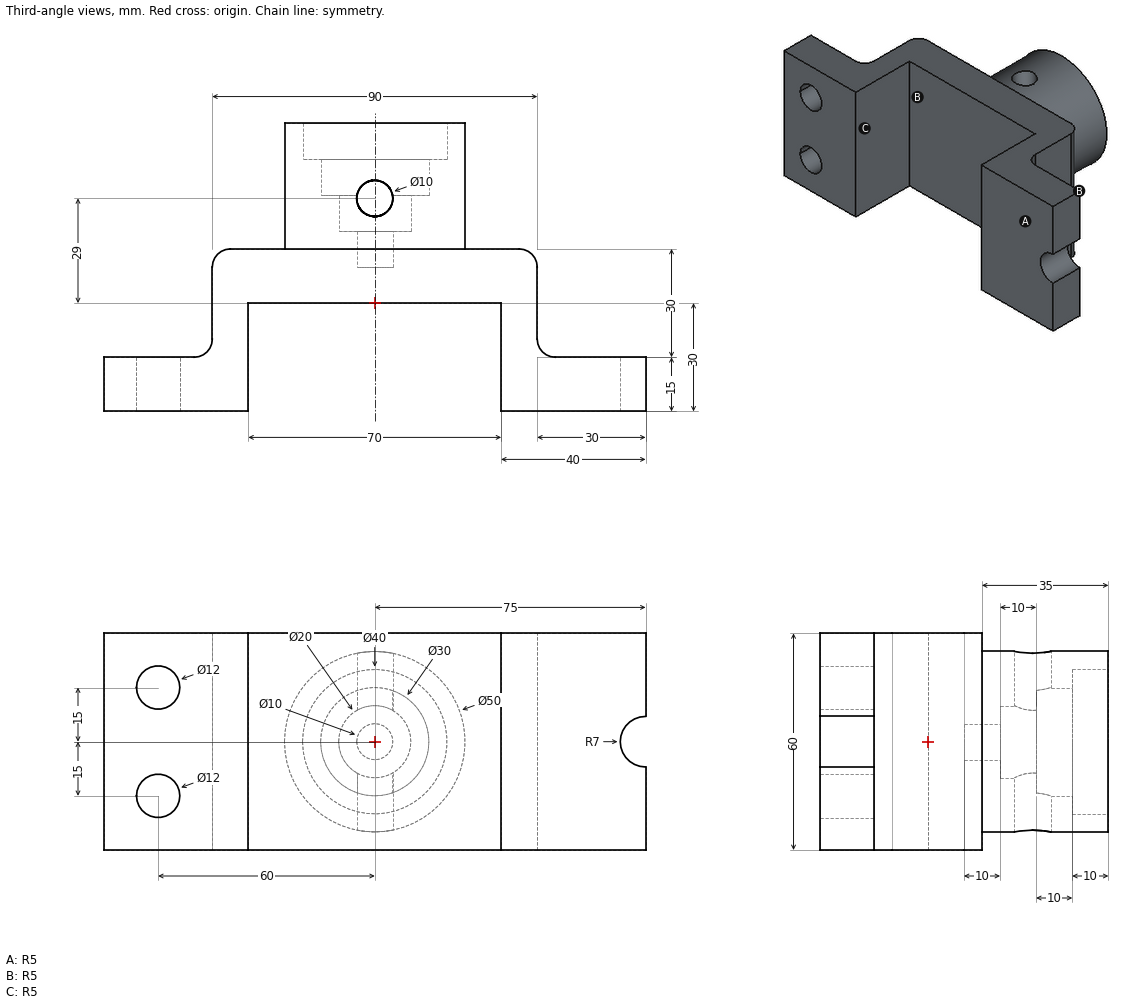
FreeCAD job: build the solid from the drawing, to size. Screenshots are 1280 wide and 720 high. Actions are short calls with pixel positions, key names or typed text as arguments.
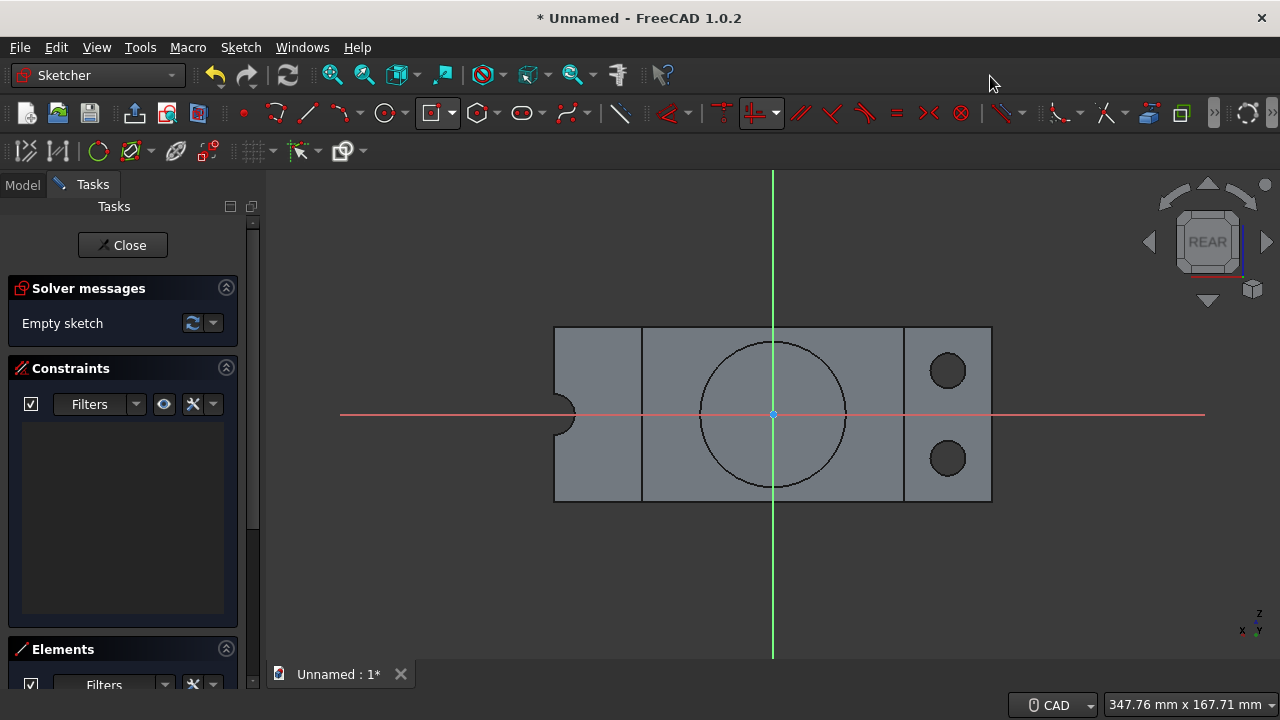
scroll(813, 415, up, 5)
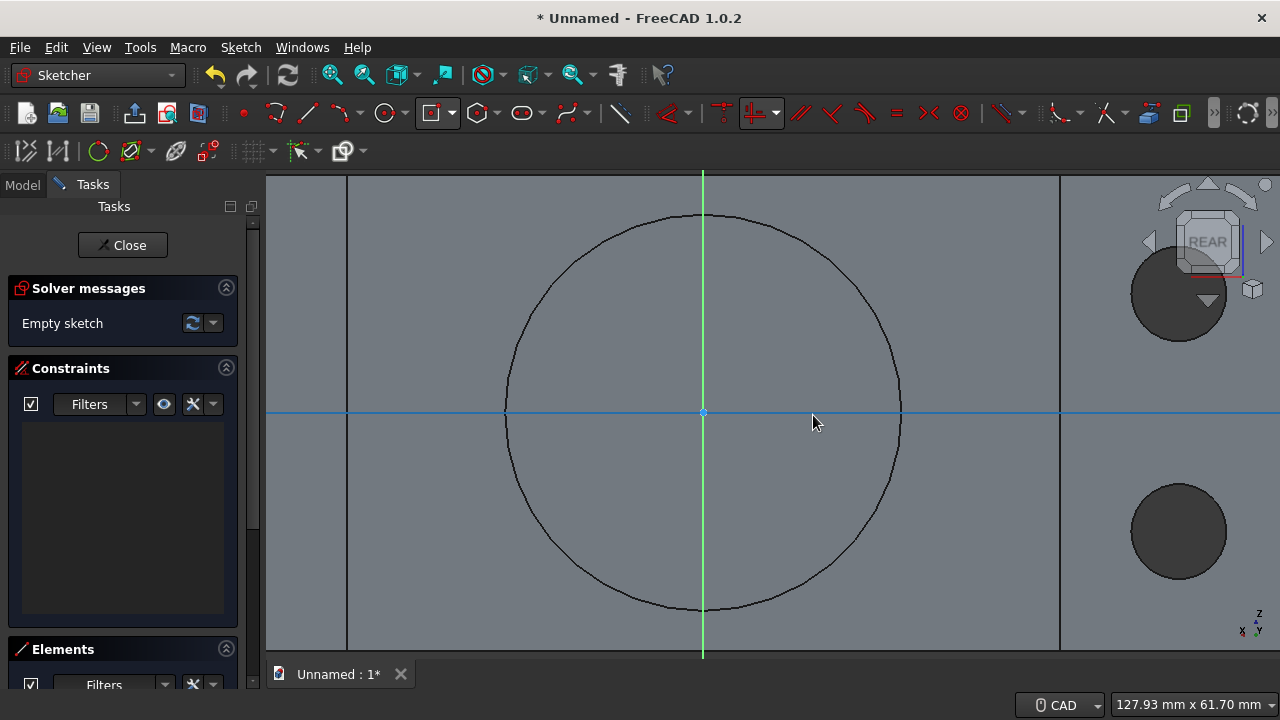
click(386, 114)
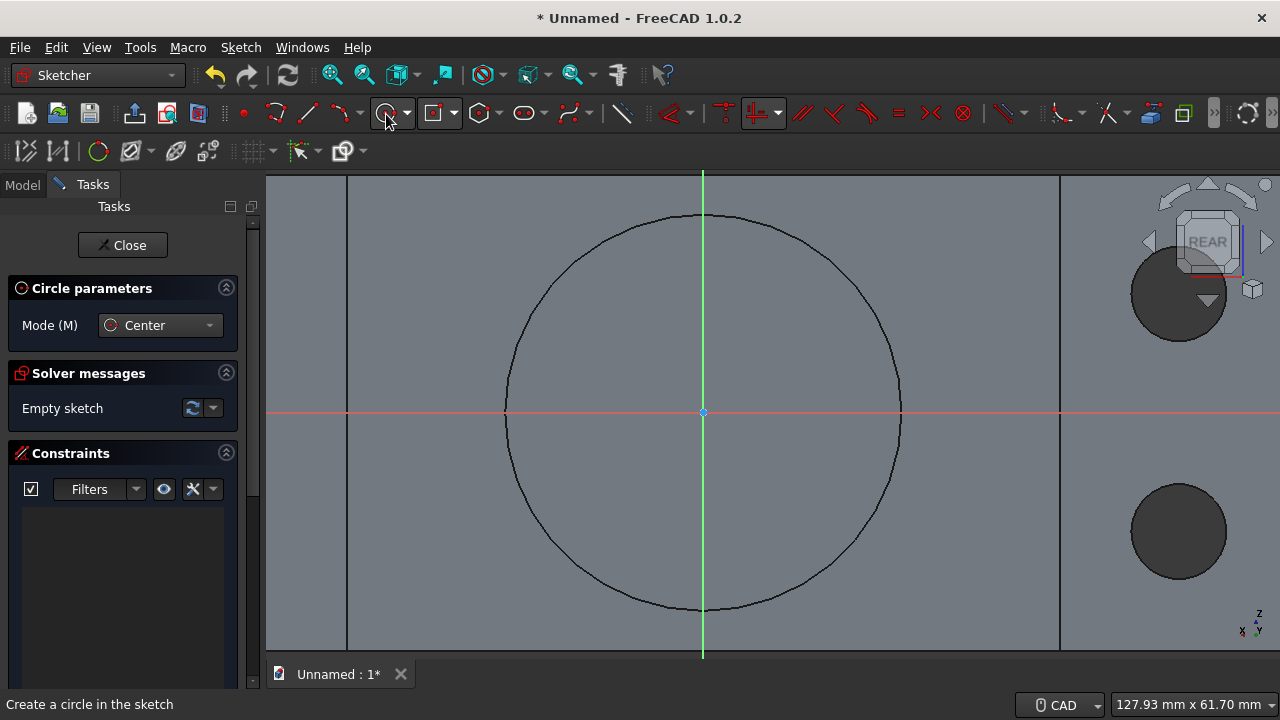
click(703, 413)
click(815, 301)
key(Escape)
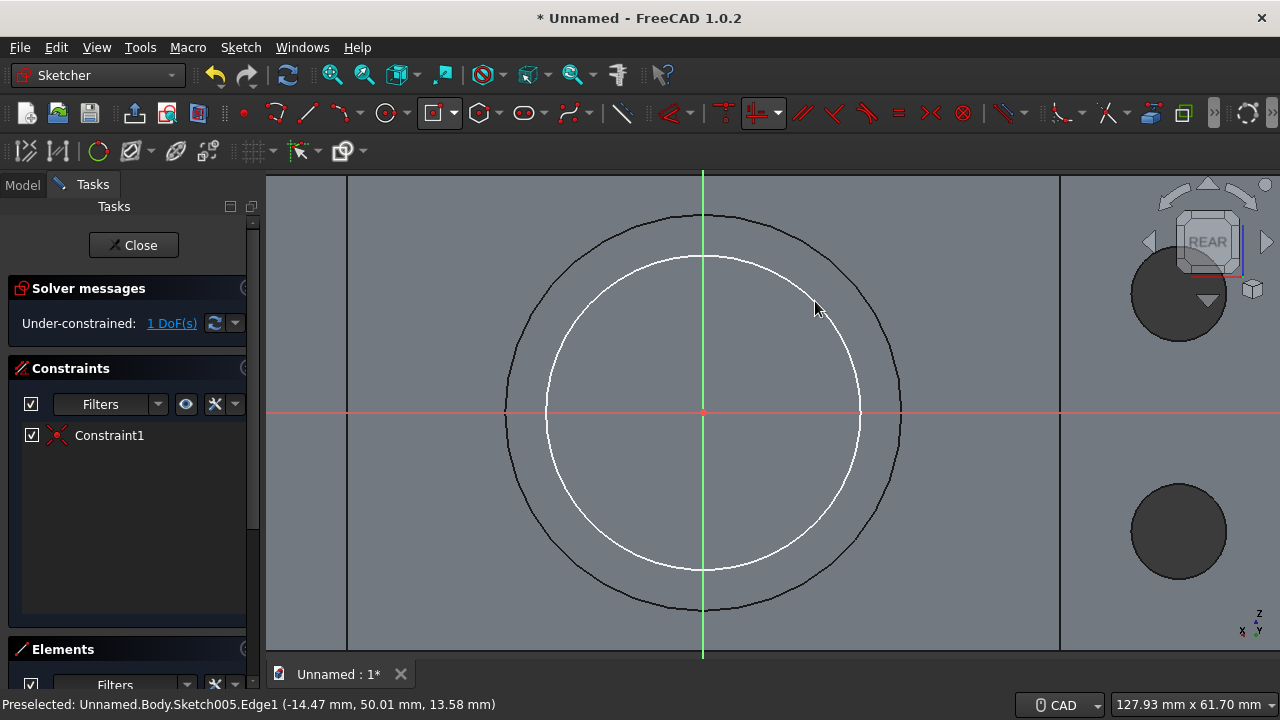
click(670, 114)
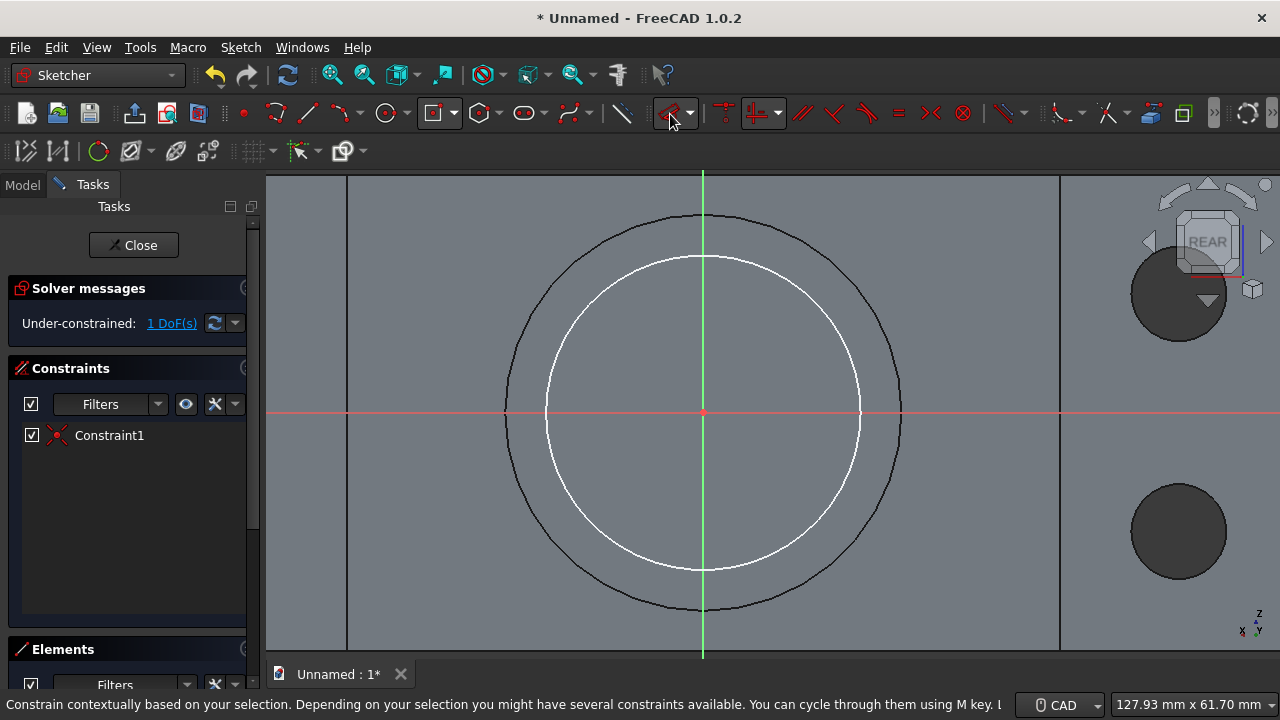
click(814, 301)
click(837, 278)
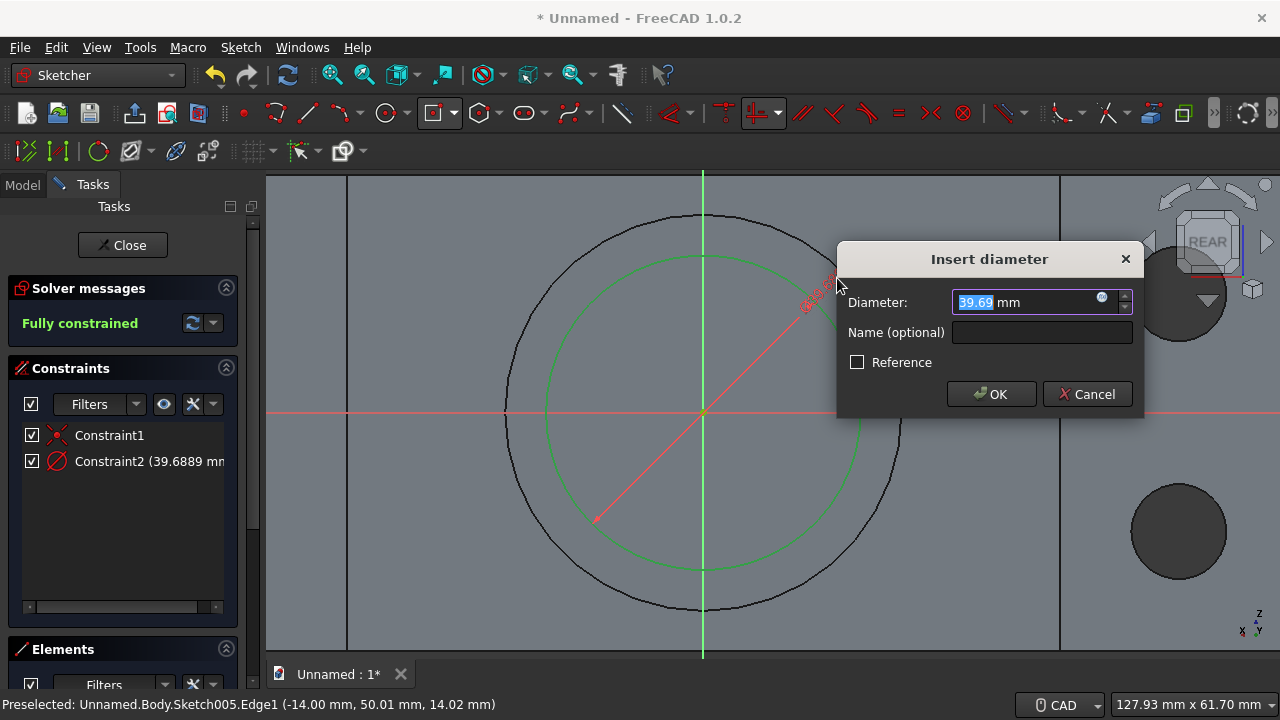
text(40)
key(Return)
key(Escape)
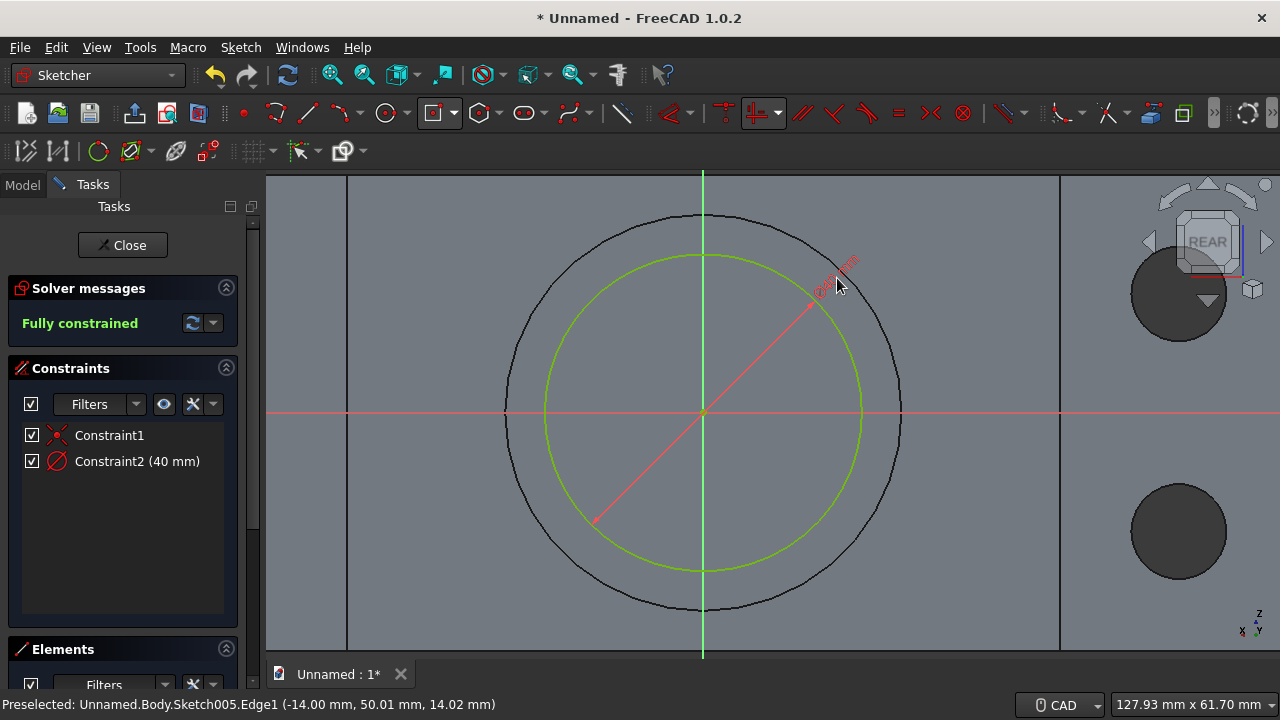
click(123, 245)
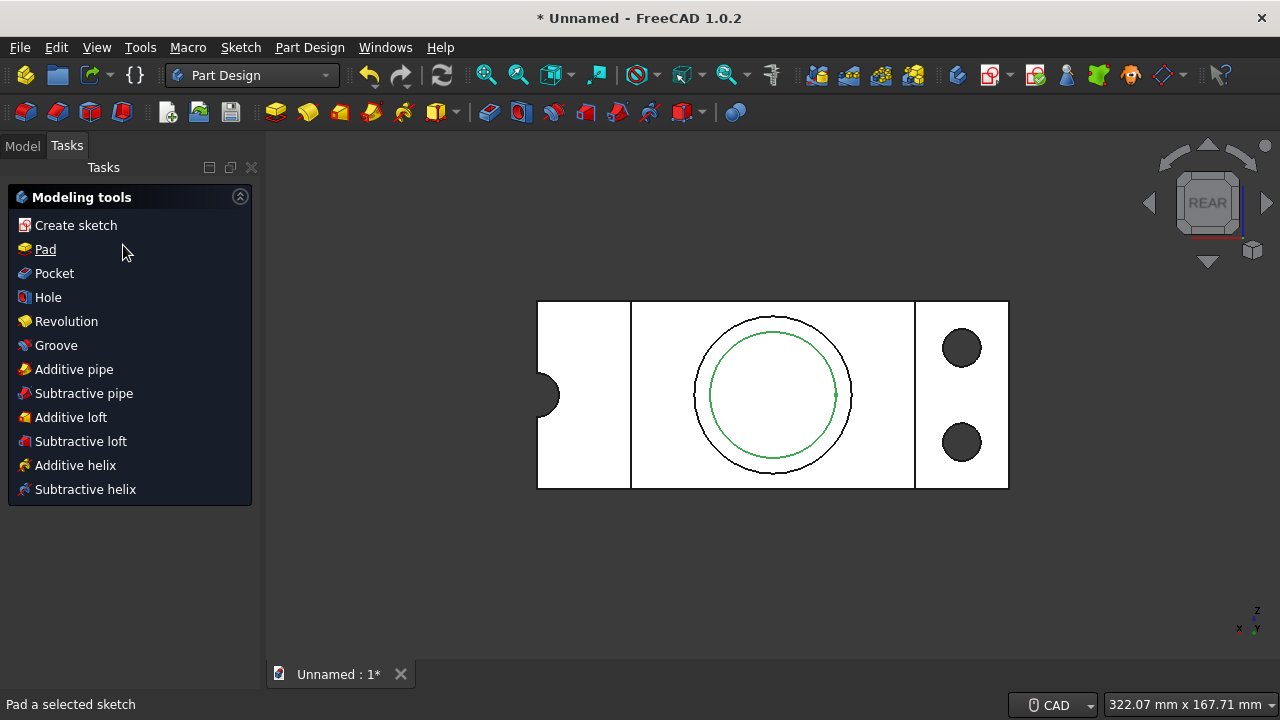
click(490, 112)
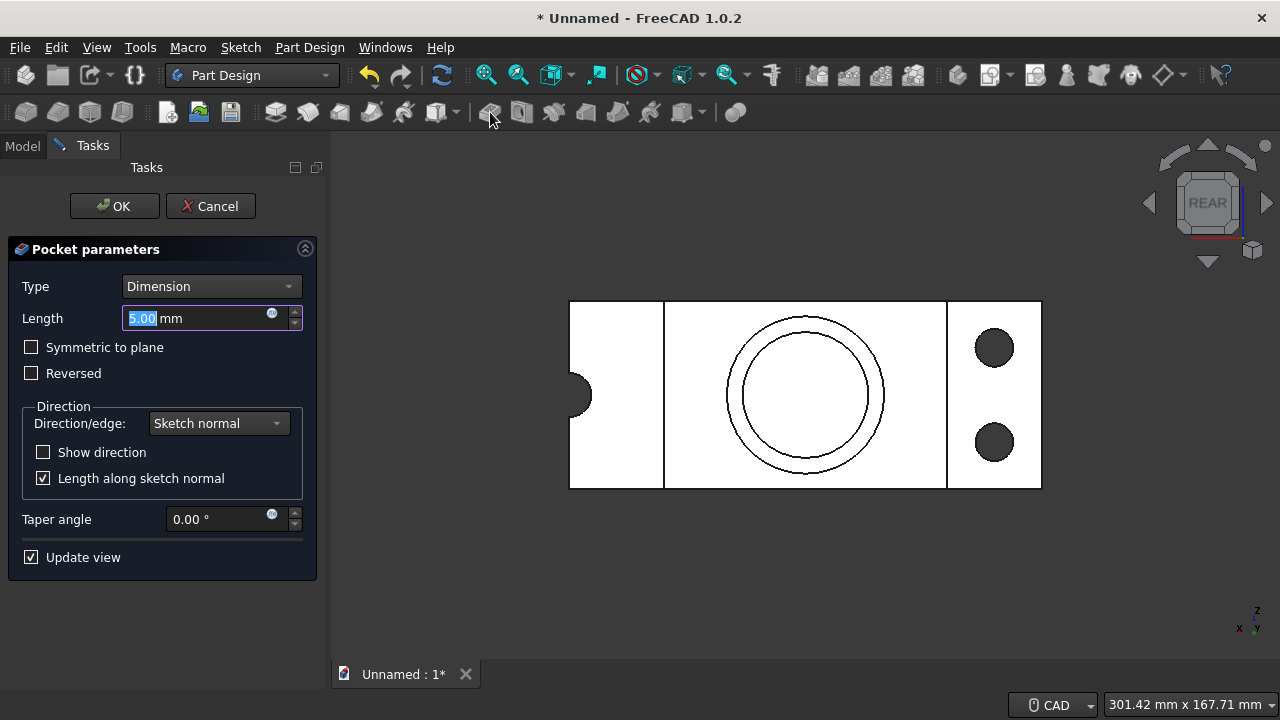
text(10)
key(Tab)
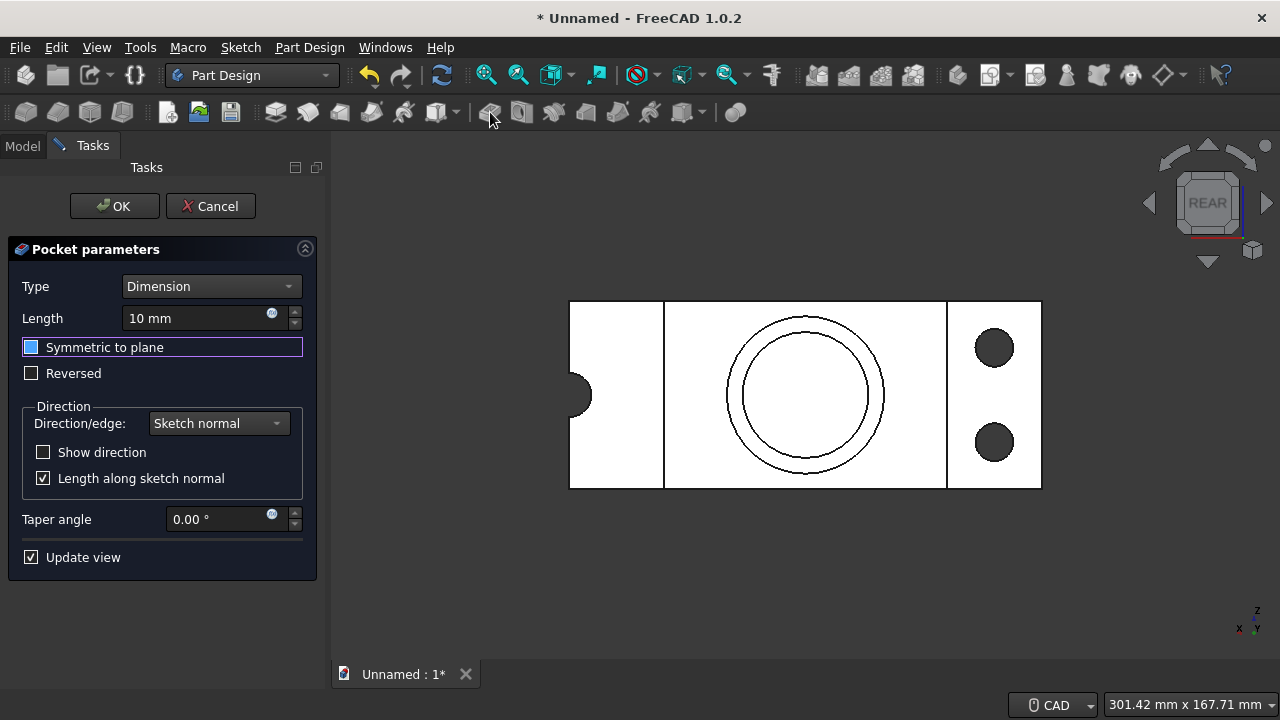
click(115, 206)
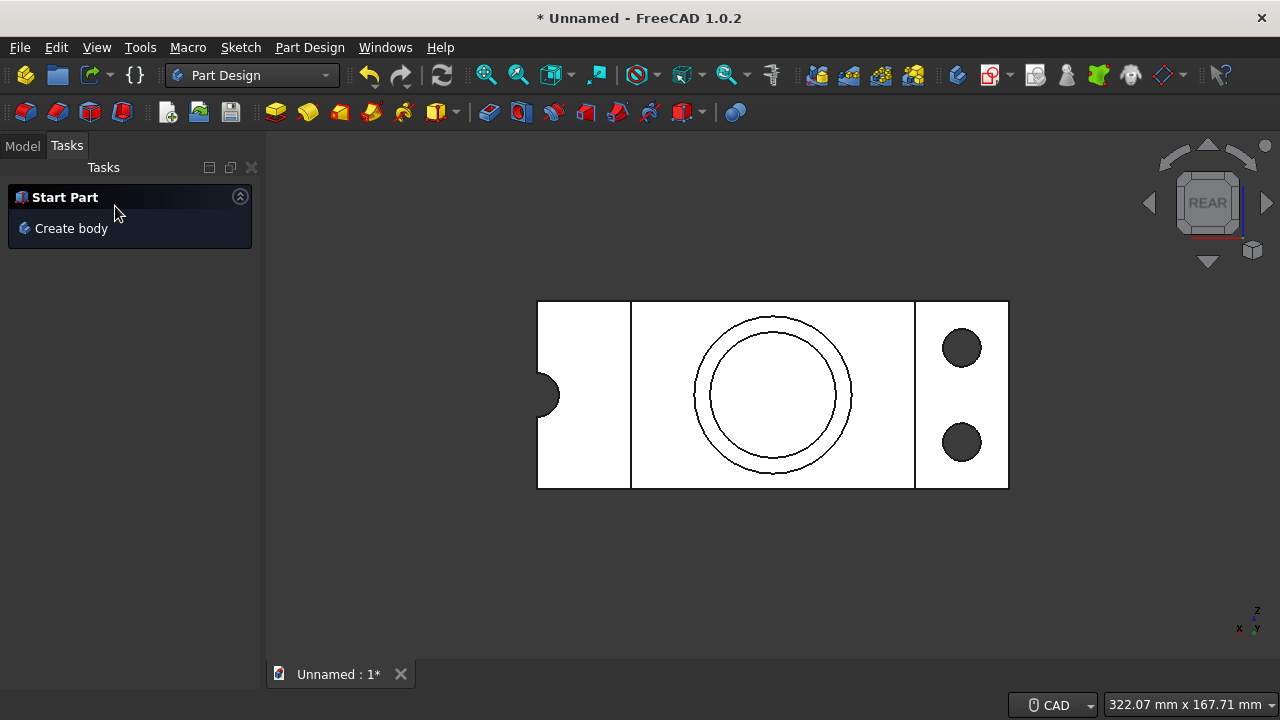
click(773, 394)